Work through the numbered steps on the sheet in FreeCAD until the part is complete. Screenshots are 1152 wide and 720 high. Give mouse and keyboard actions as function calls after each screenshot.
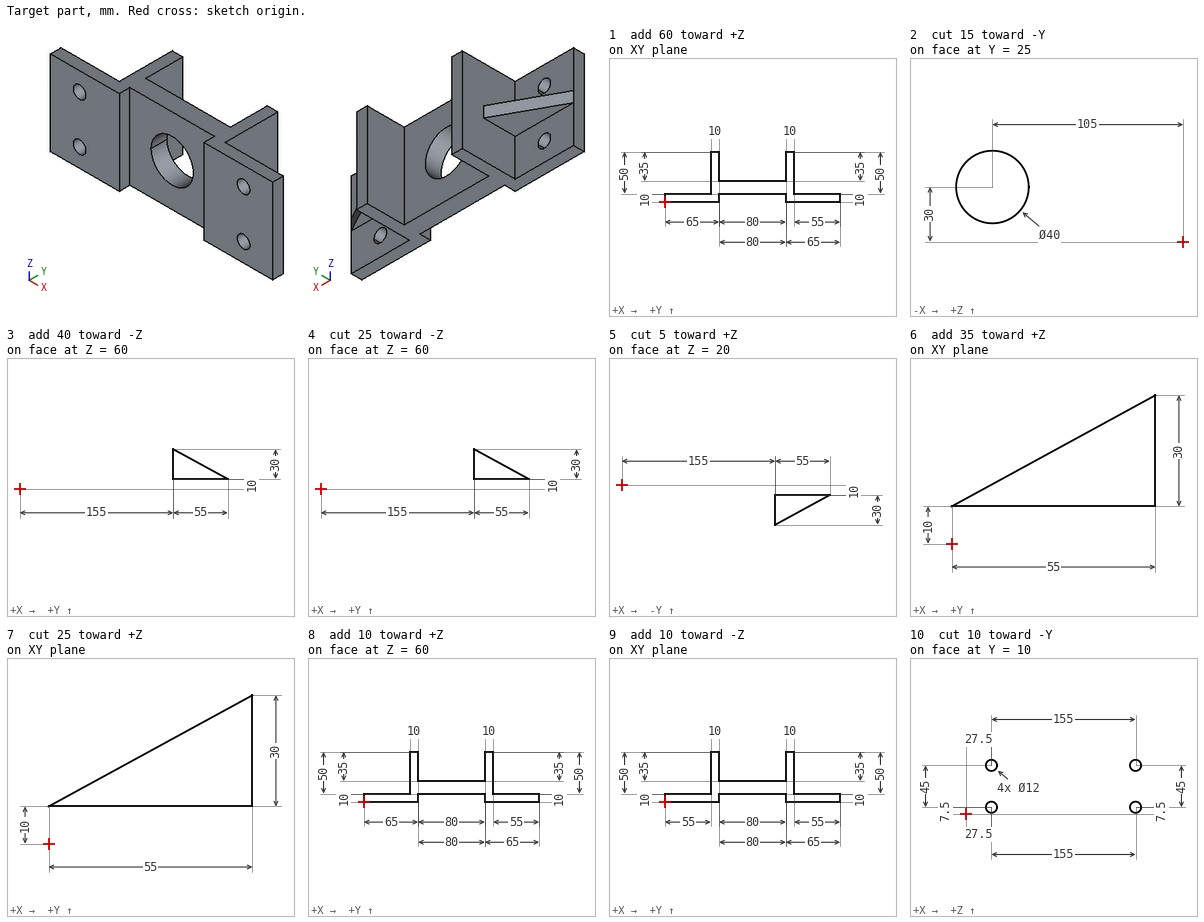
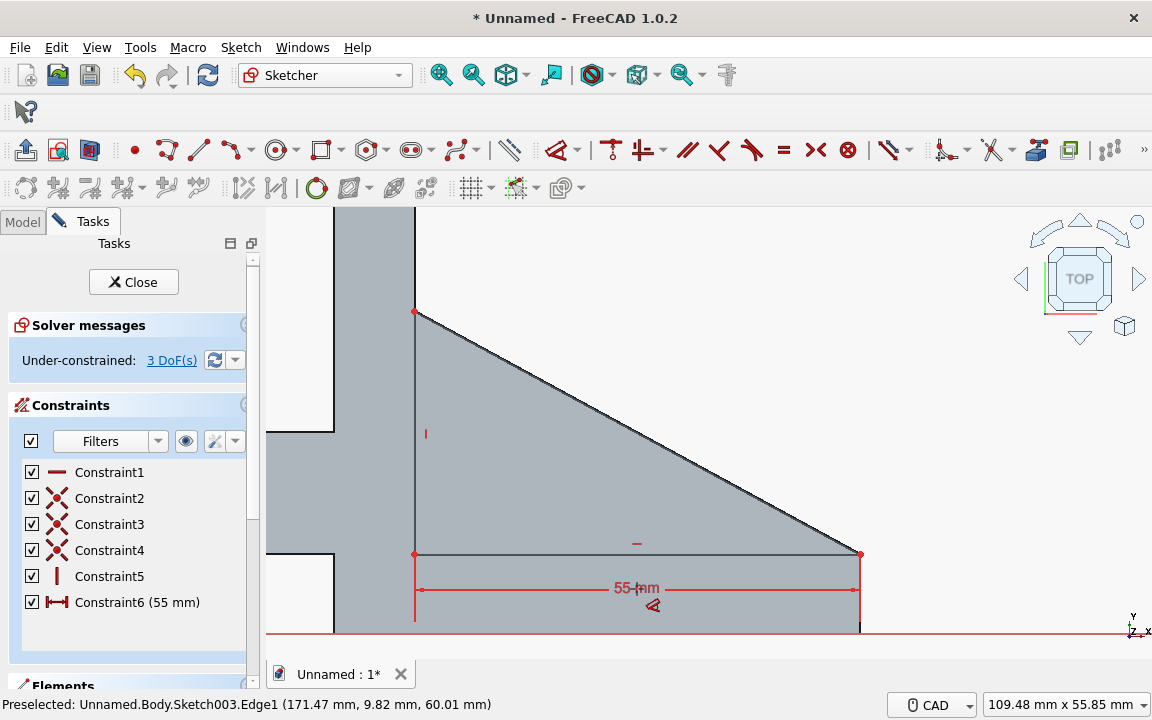
click(415, 385)
click(381, 433)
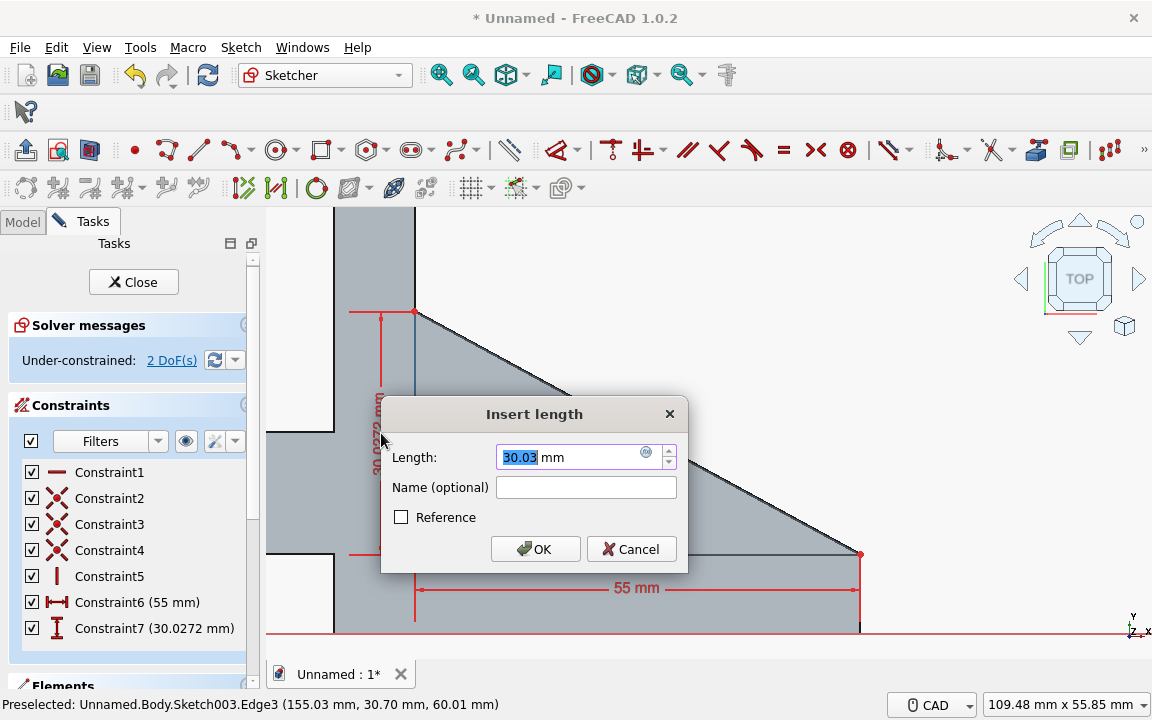
text(30)
key(Return)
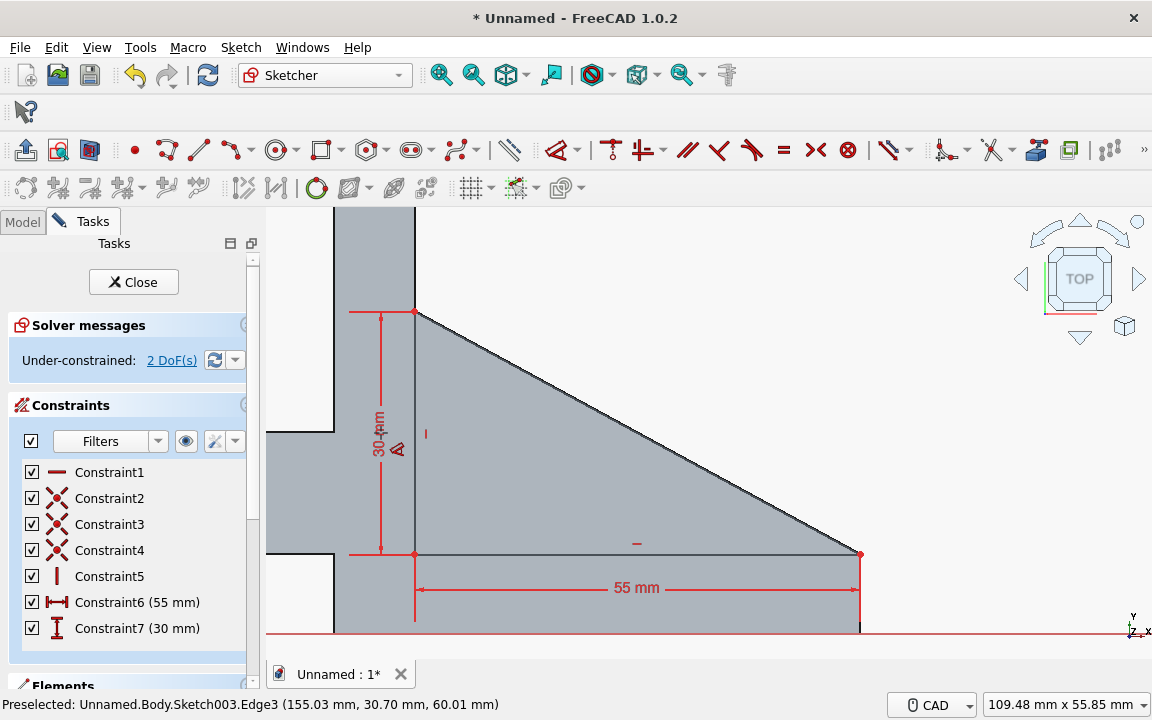
click(415, 555)
click(449, 593)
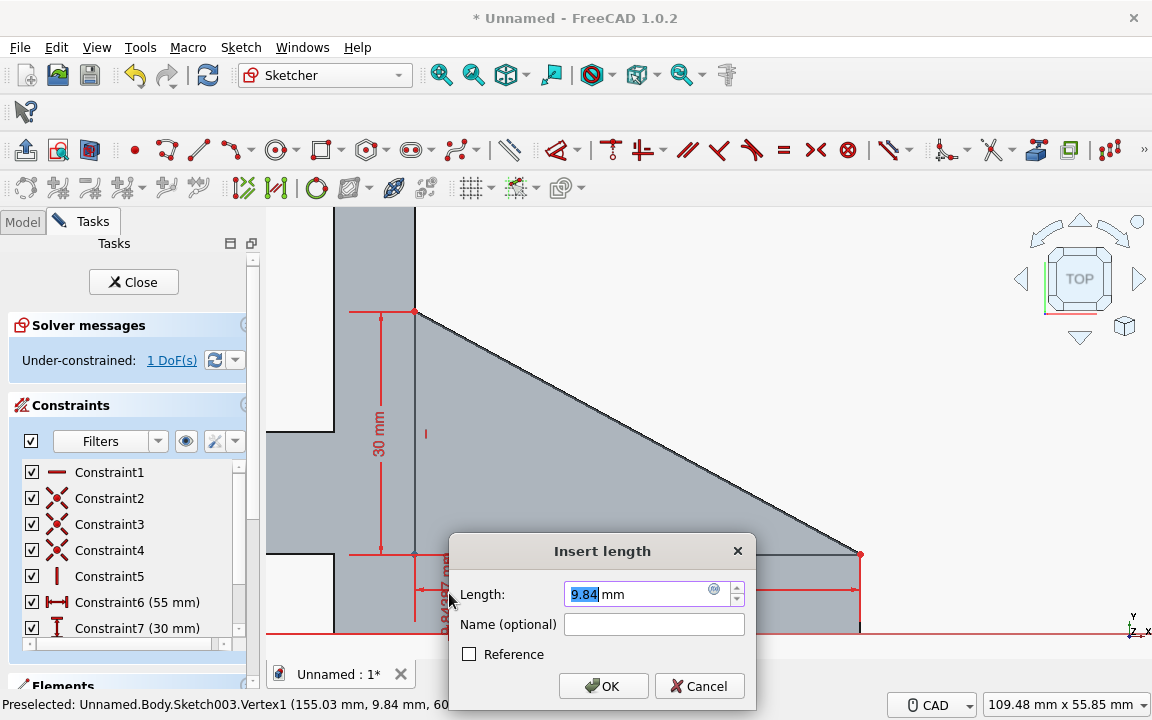
text(10)
key(Return)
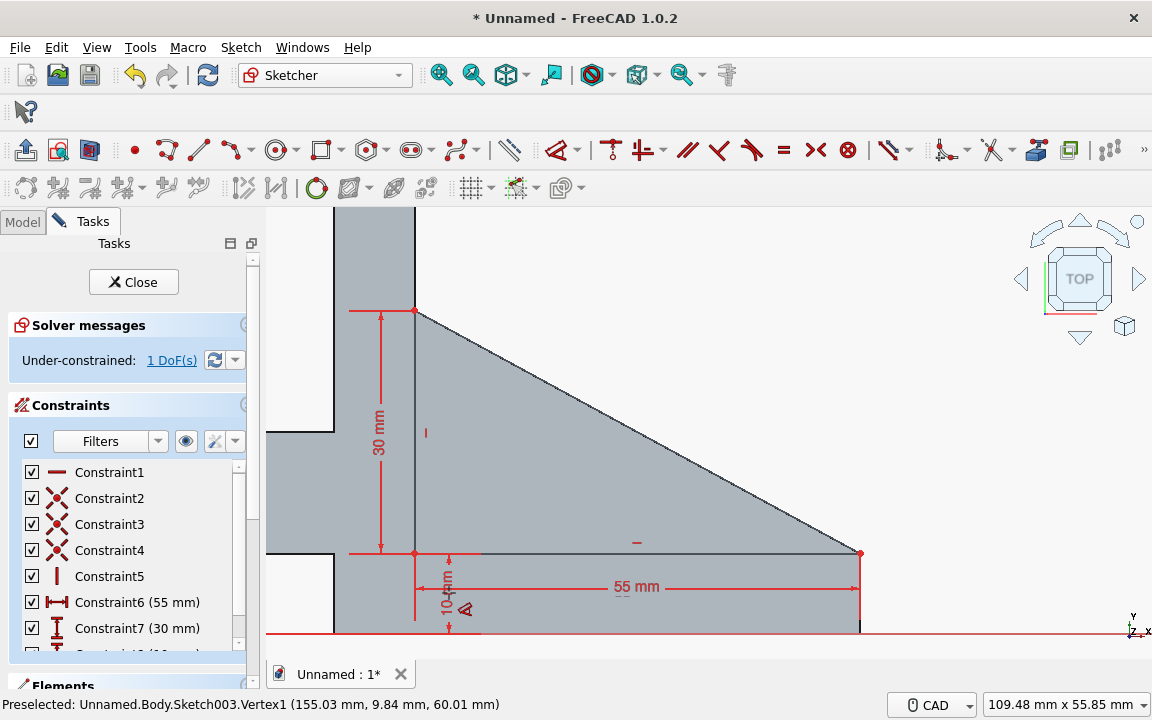
click(415, 554)
click(354, 520)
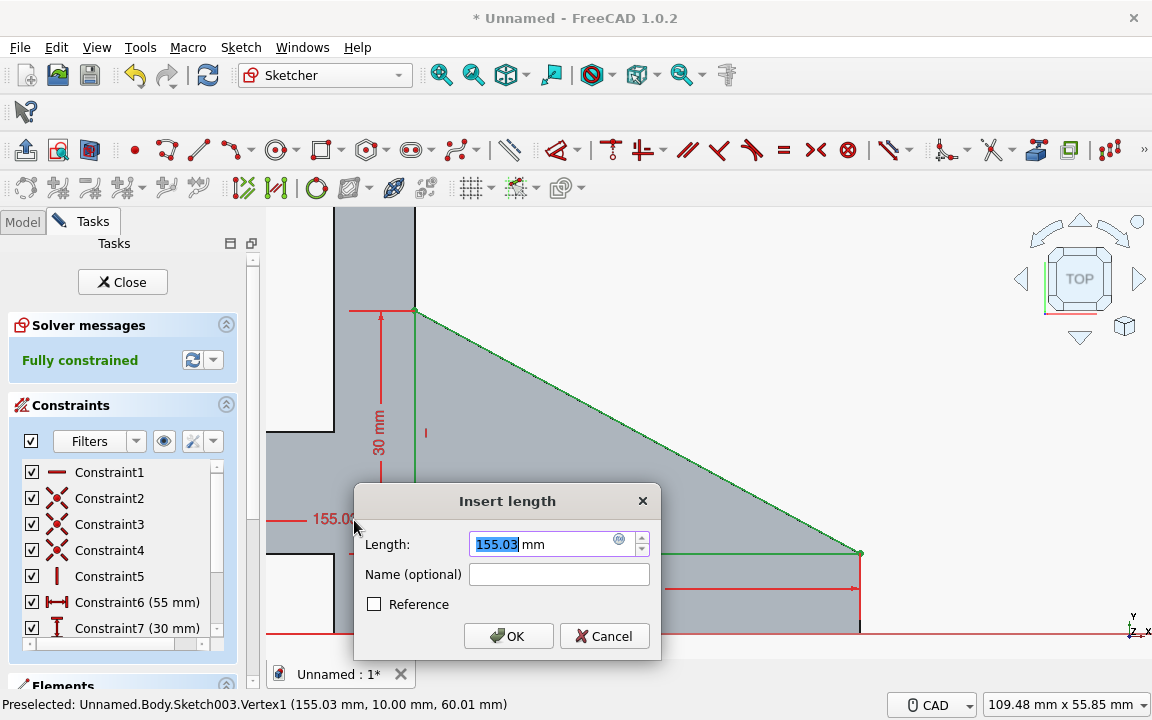
text(155)
key(Return)
key(Escape)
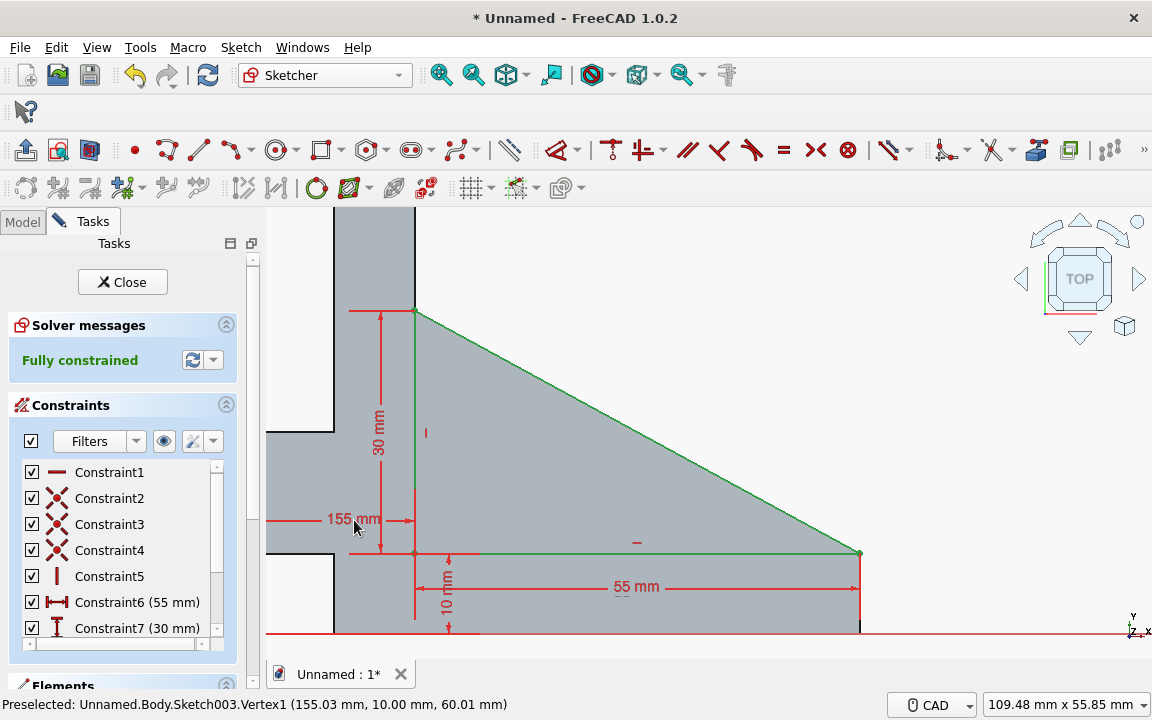
click(123, 282)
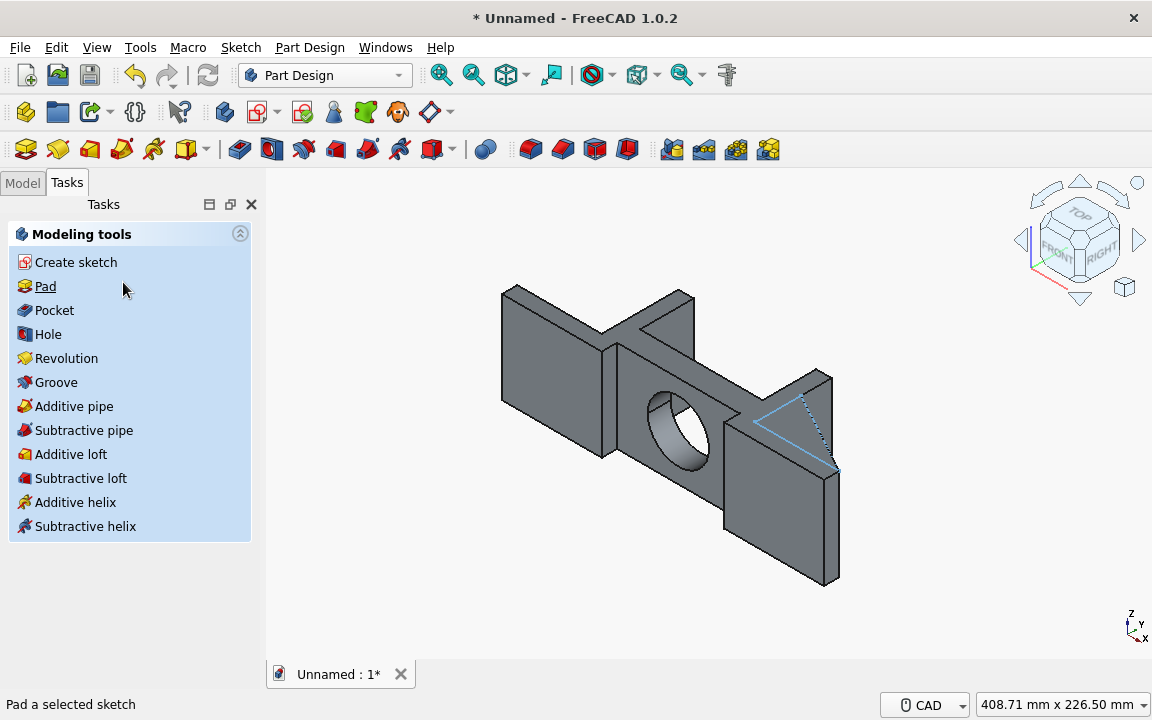
click(240, 150)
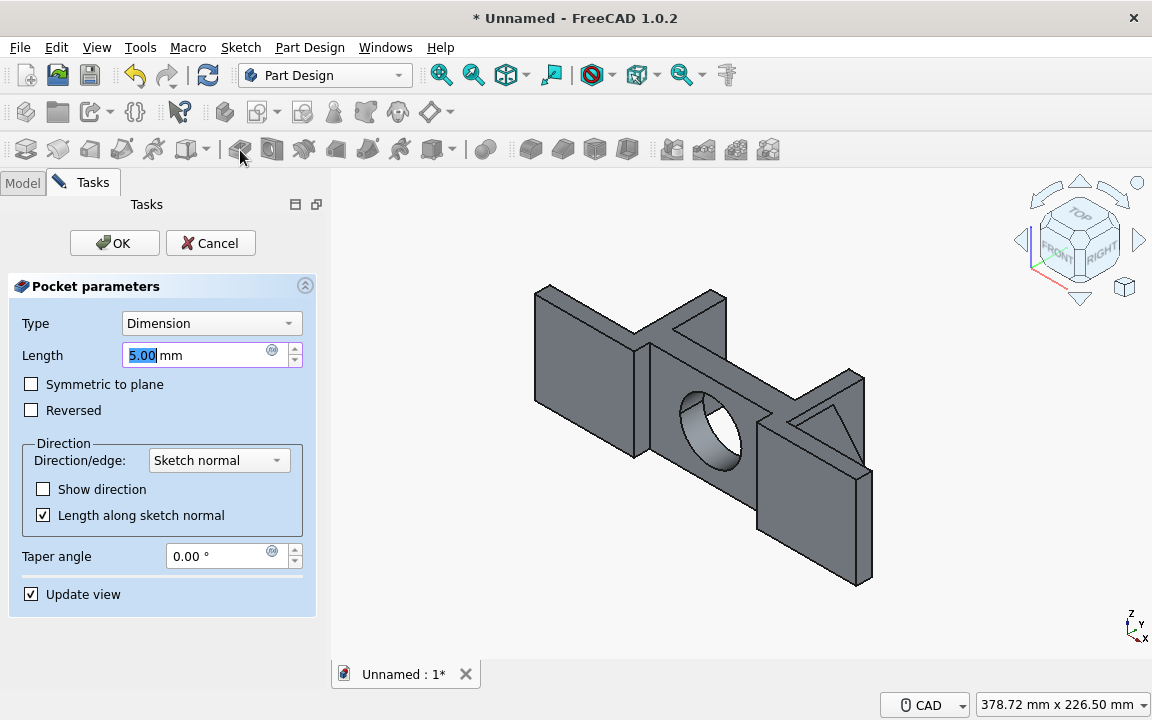
text(25)
key(Tab)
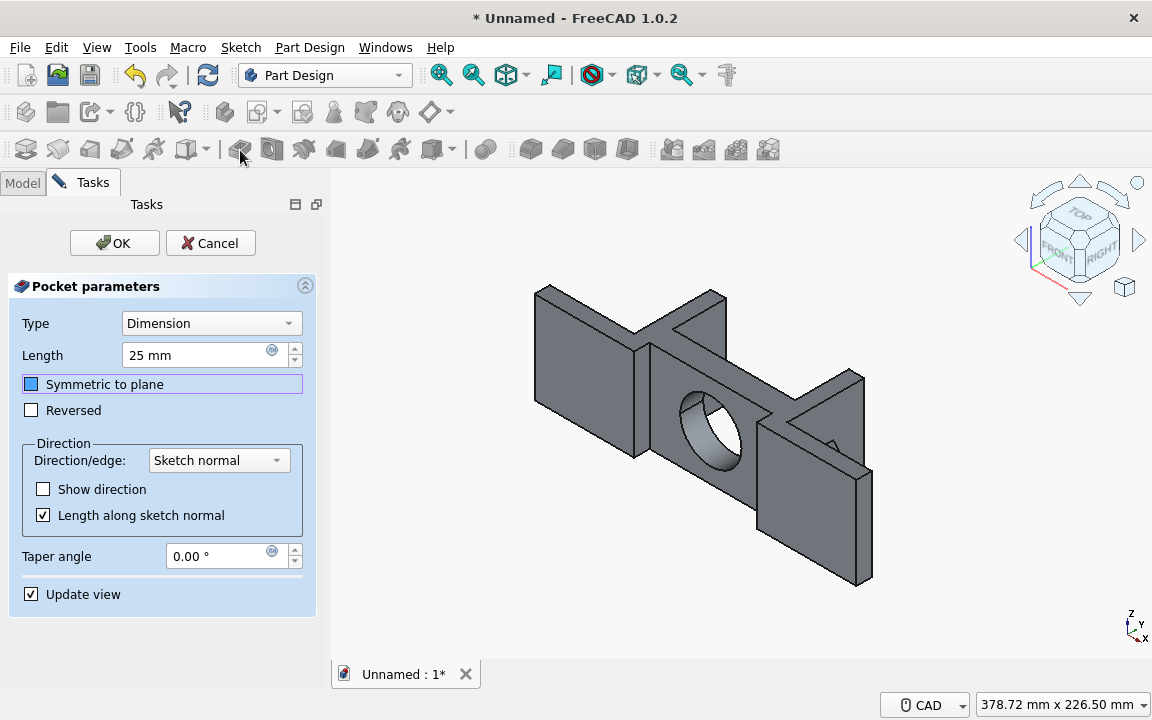
click(115, 243)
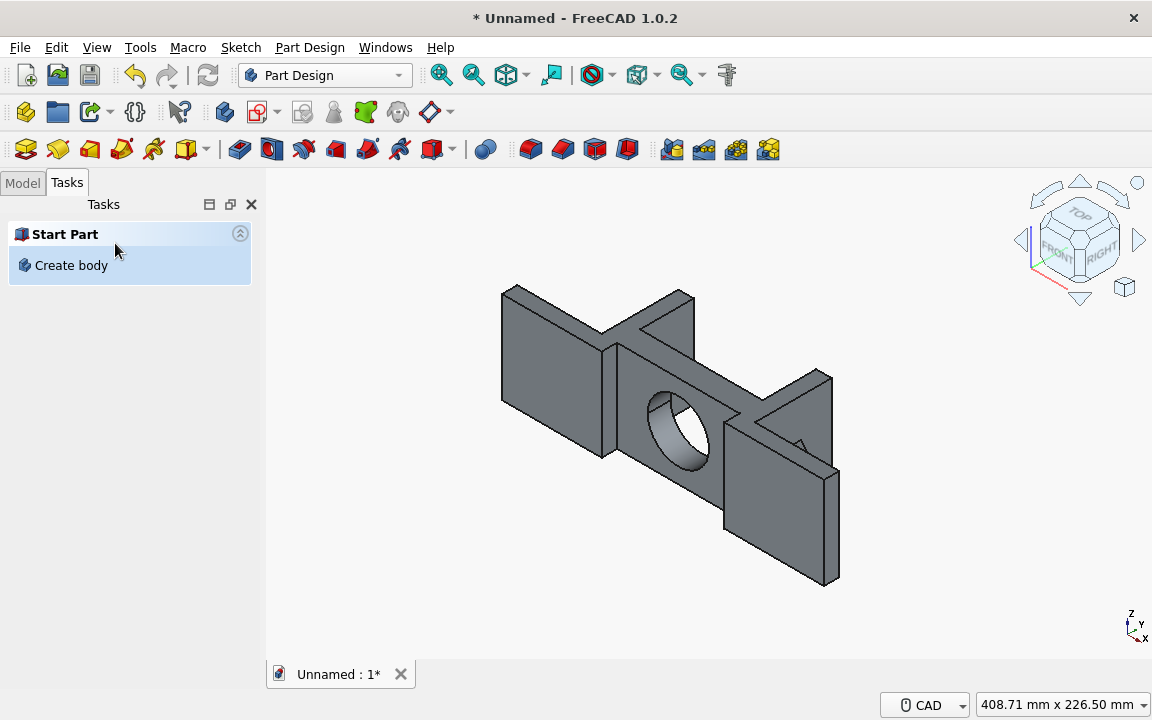
key(5)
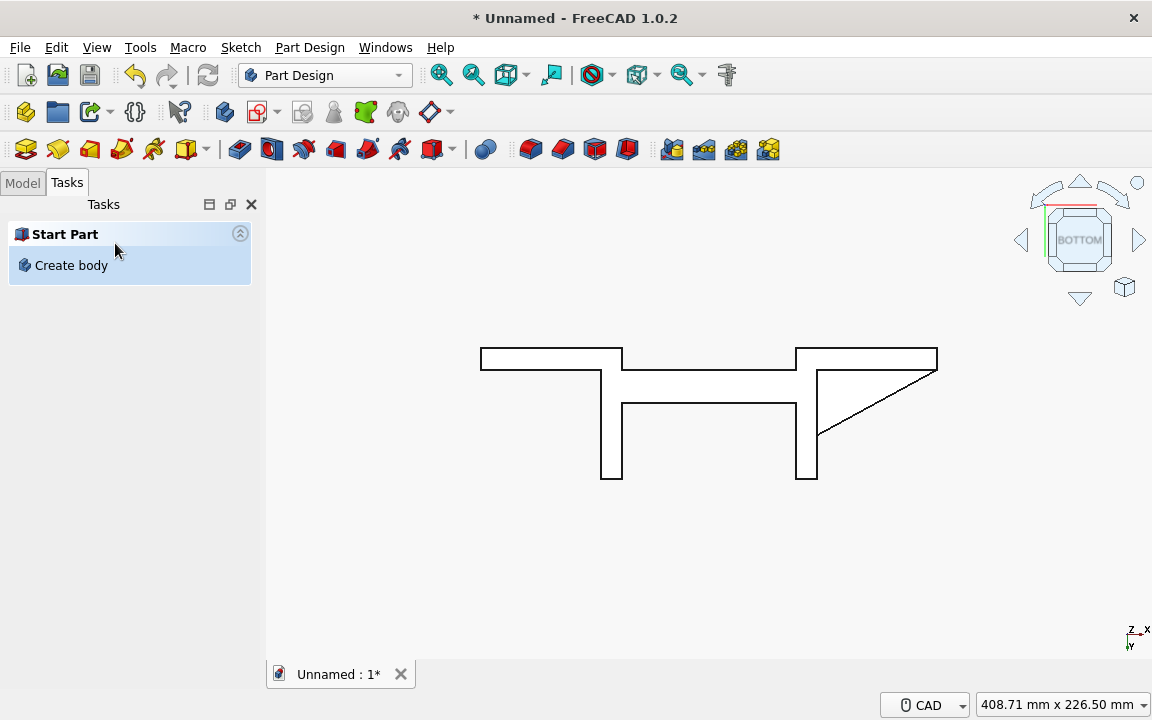
click(843, 392)